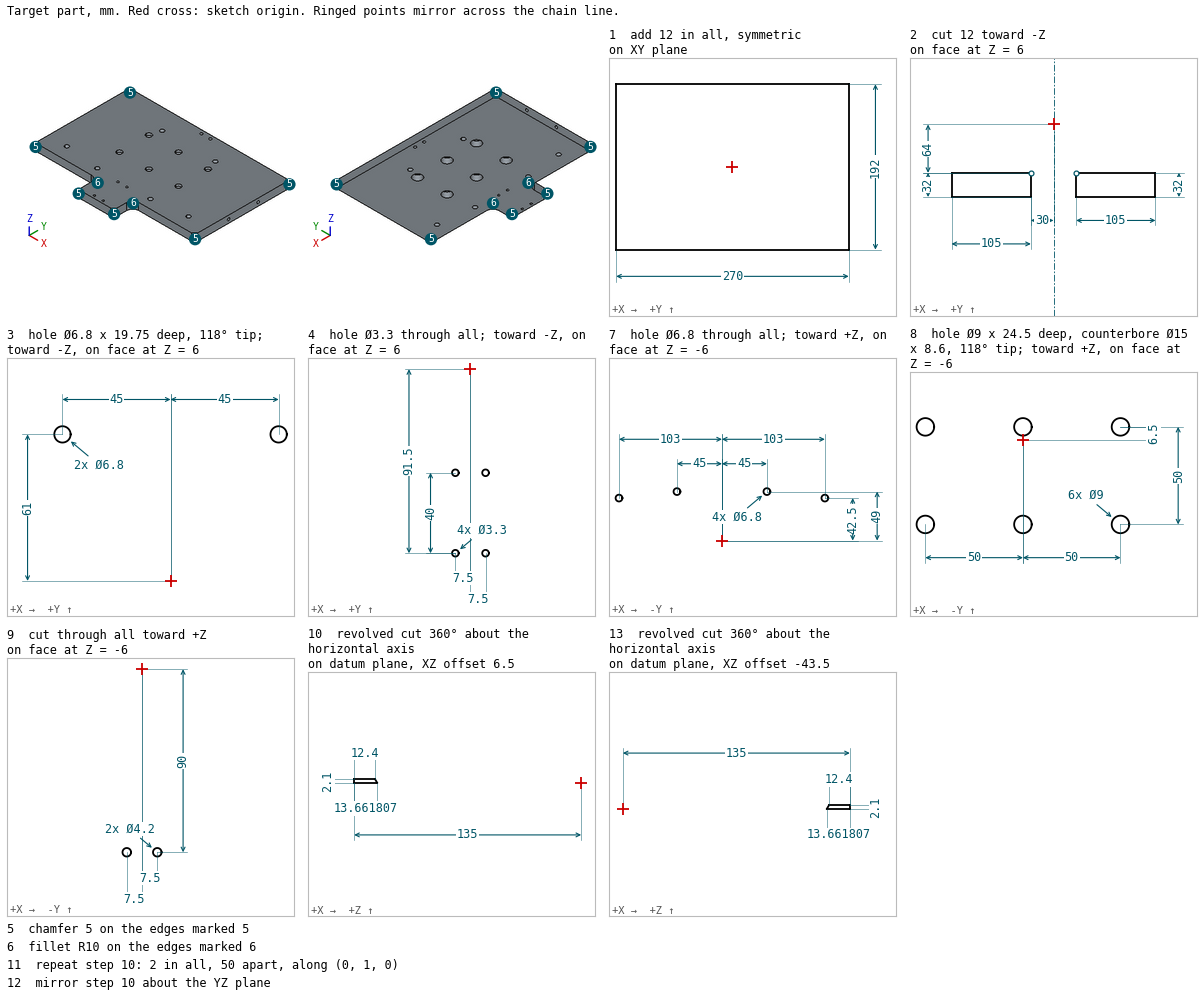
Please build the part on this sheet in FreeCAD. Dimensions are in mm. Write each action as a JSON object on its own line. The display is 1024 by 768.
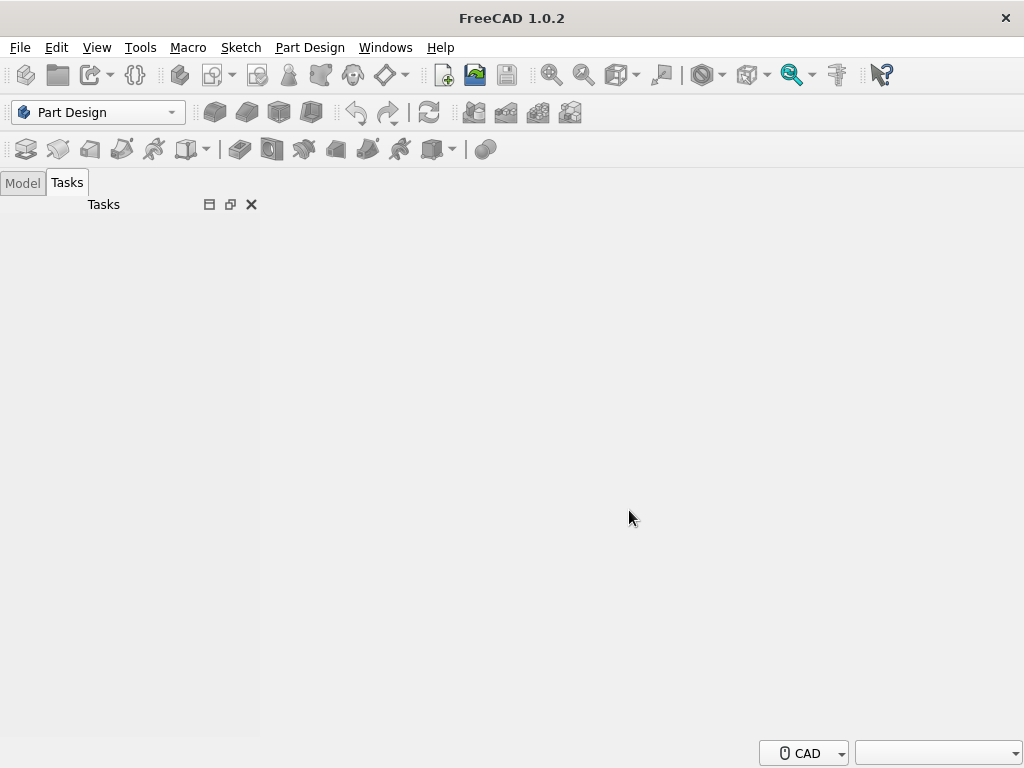
{"action": "key", "text": "ctrl+n"}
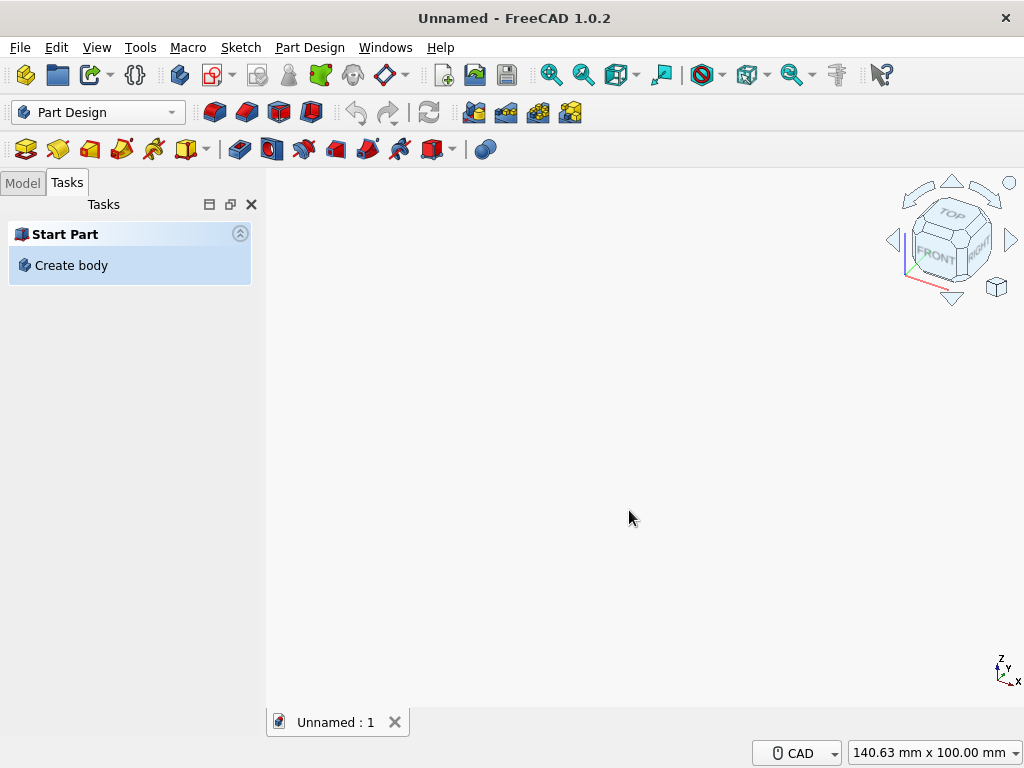
{"action": "left_click", "coordinate": [212, 76]}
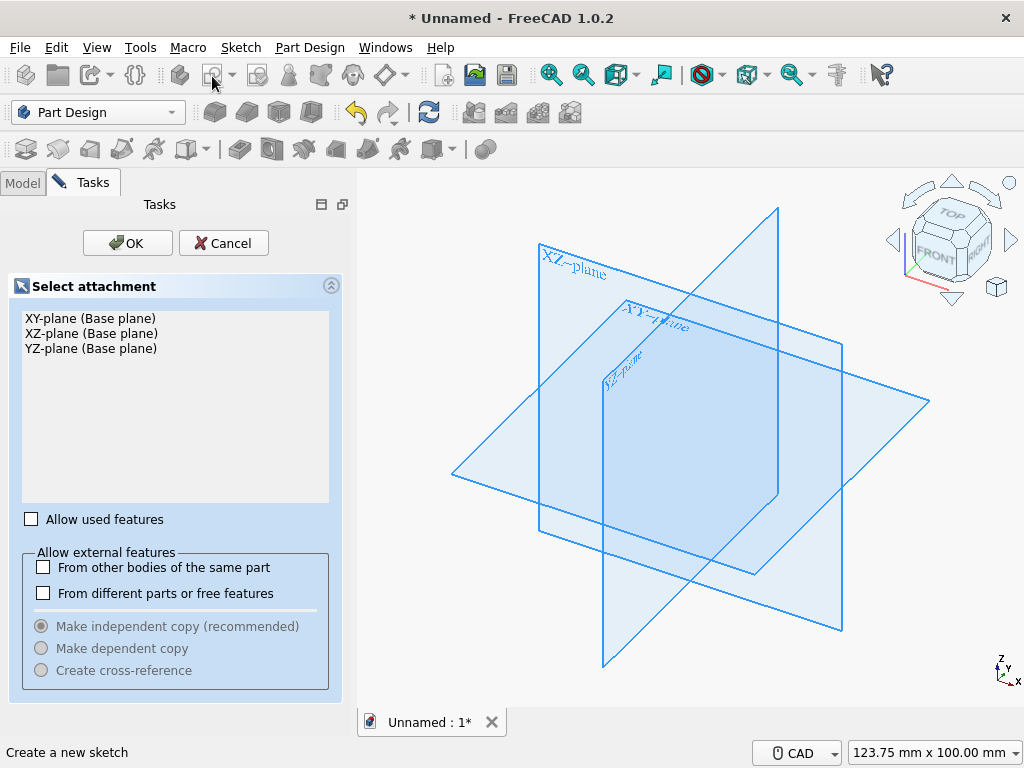
{"action": "left_click", "coordinate": [82, 318]}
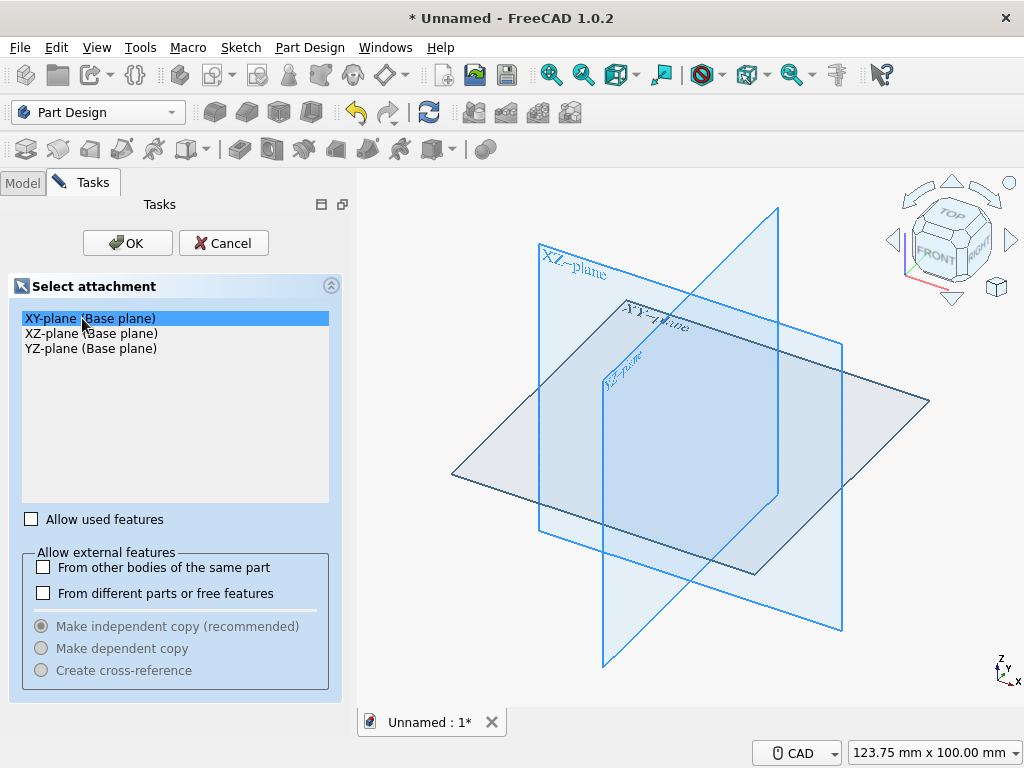
{"action": "left_click", "coordinate": [128, 243]}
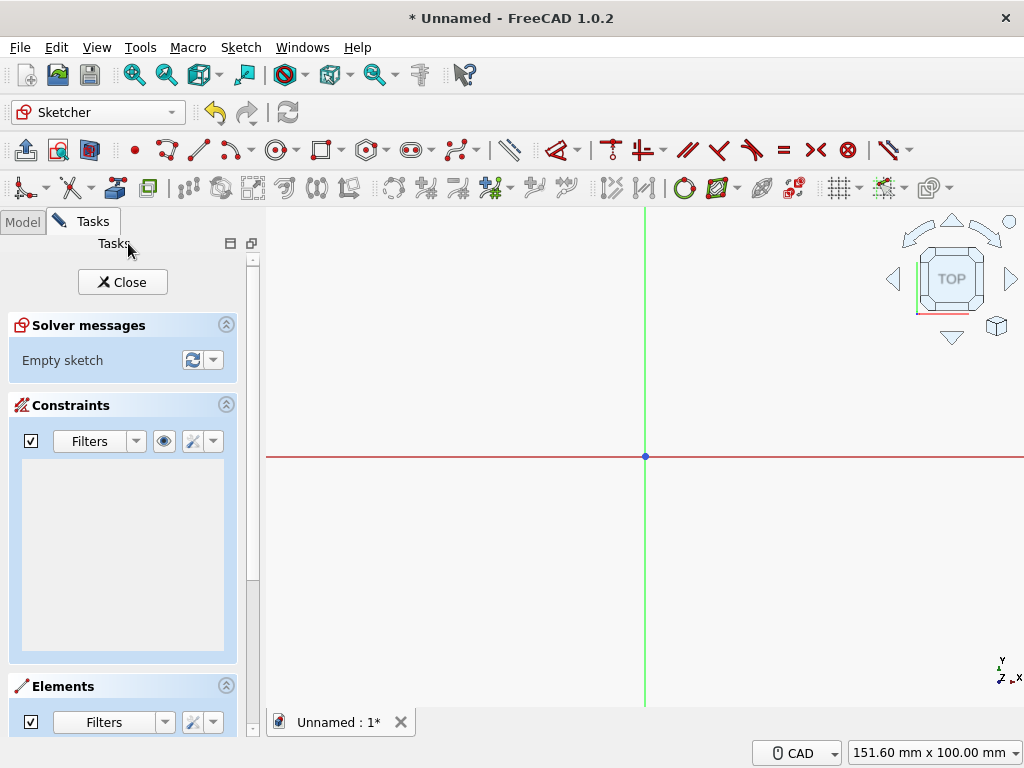
{"action": "scroll", "coordinate": [547, 457], "scroll_direction": "down", "scroll_amount": 6}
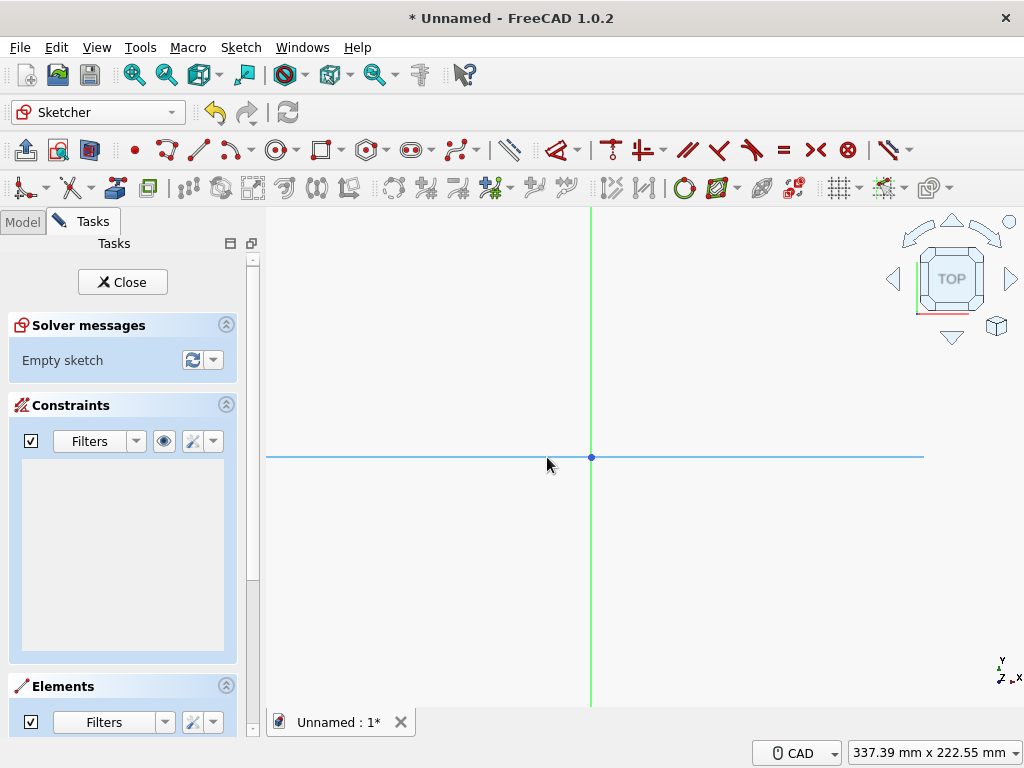
{"action": "key", "text": "g v"}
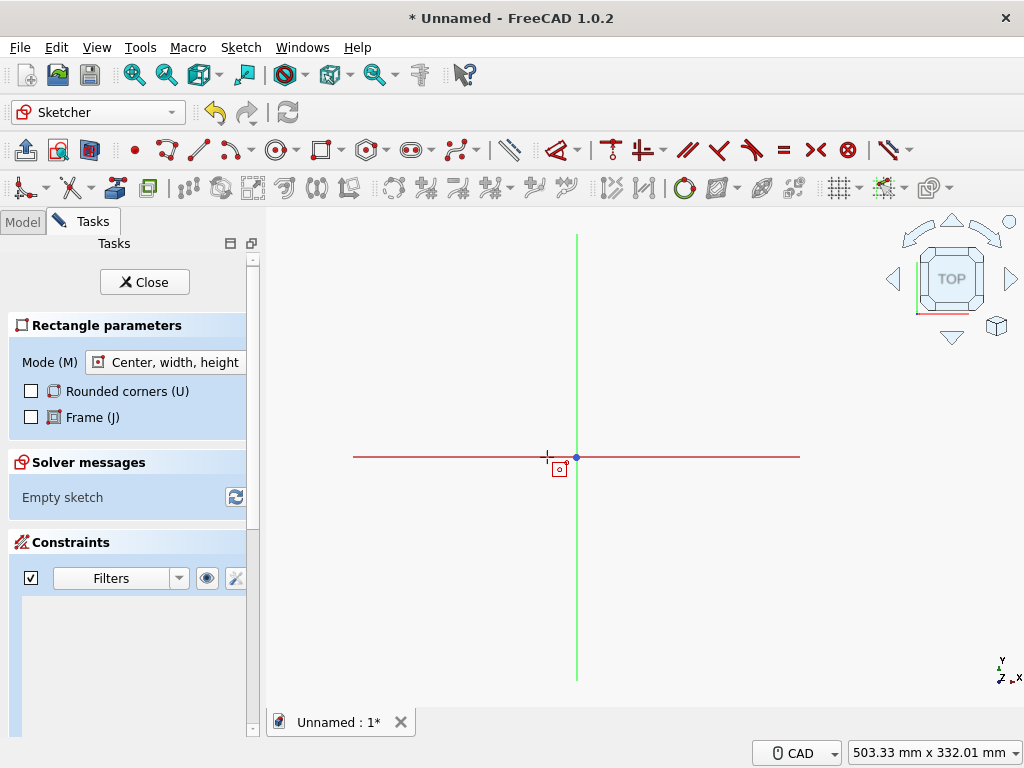
{"action": "left_click", "coordinate": [577, 457]}
{"action": "mouse_move", "coordinate": [780, 313]}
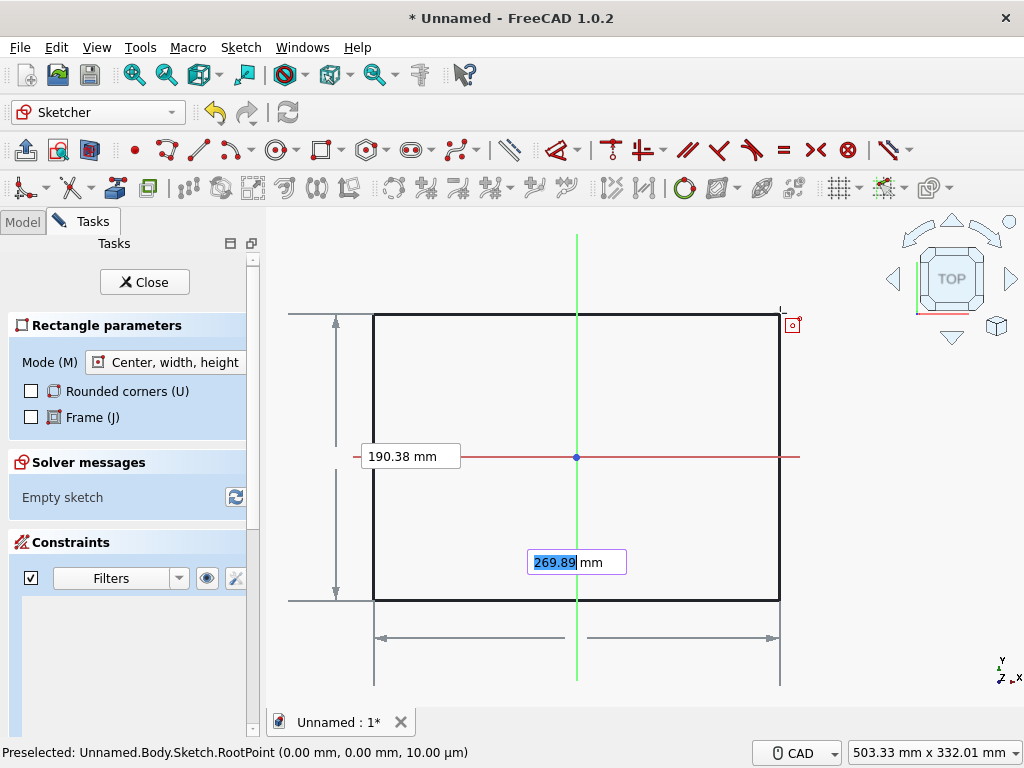
{"action": "type", "text": "270"}
{"action": "key", "text": "Tab"}
{"action": "type", "text": "192"}
{"action": "key", "text": "Return"}
{"action": "key", "text": "Escape"}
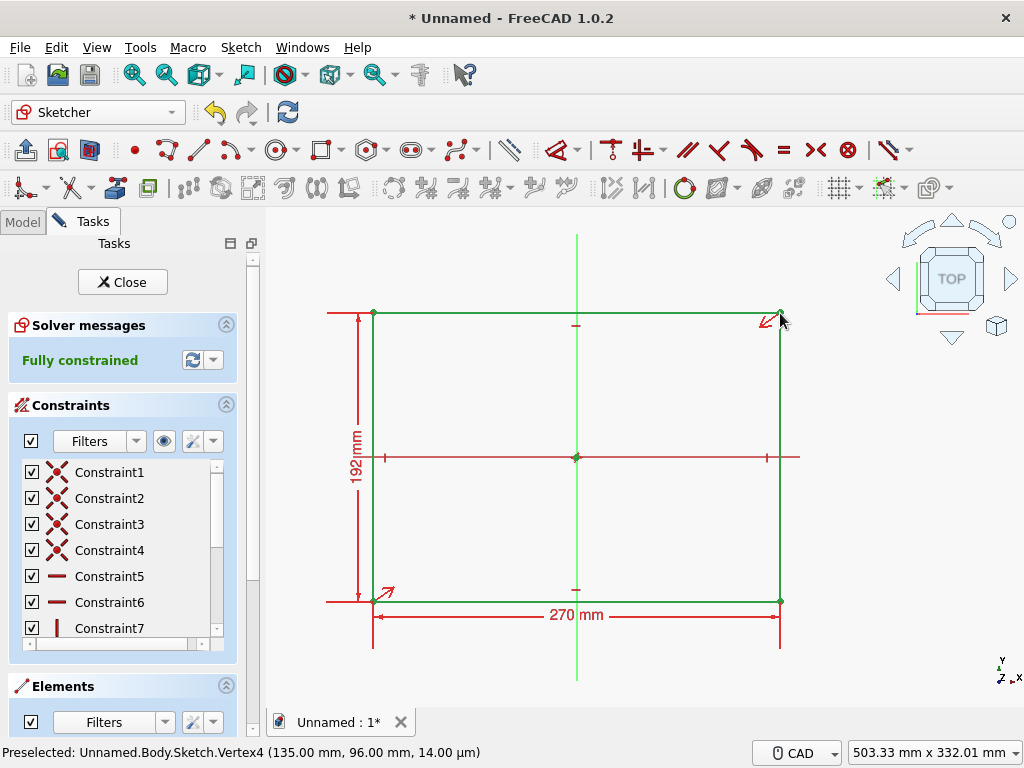
{"action": "left_click", "coordinate": [123, 282]}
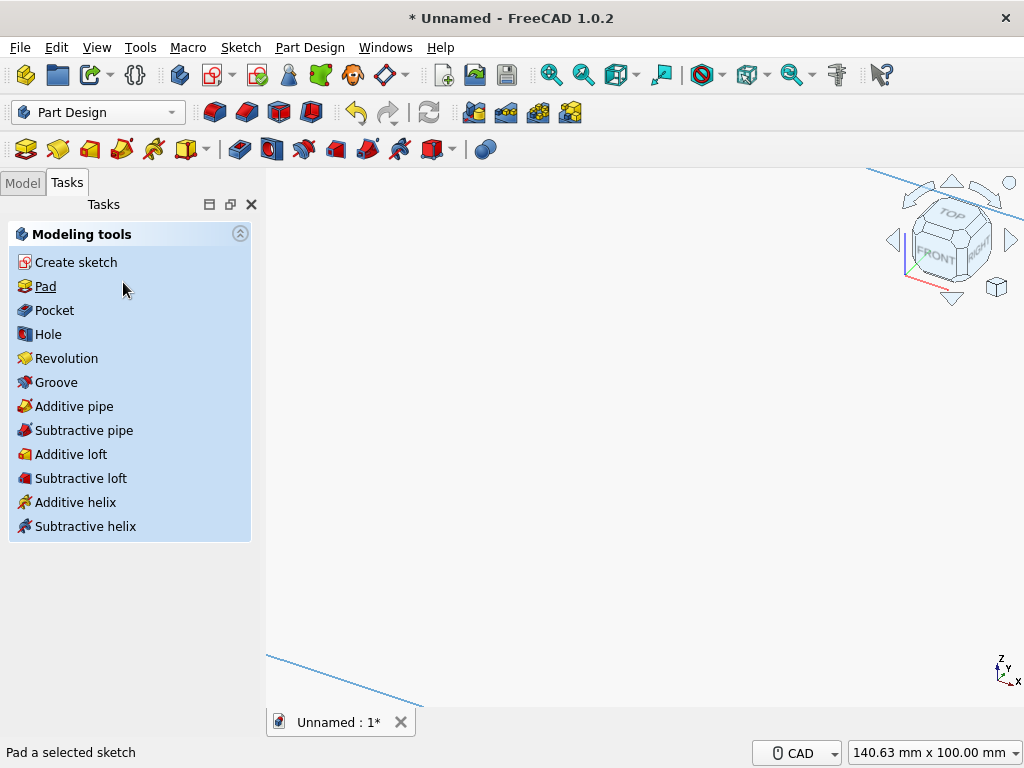
{"action": "left_click", "coordinate": [26, 150]}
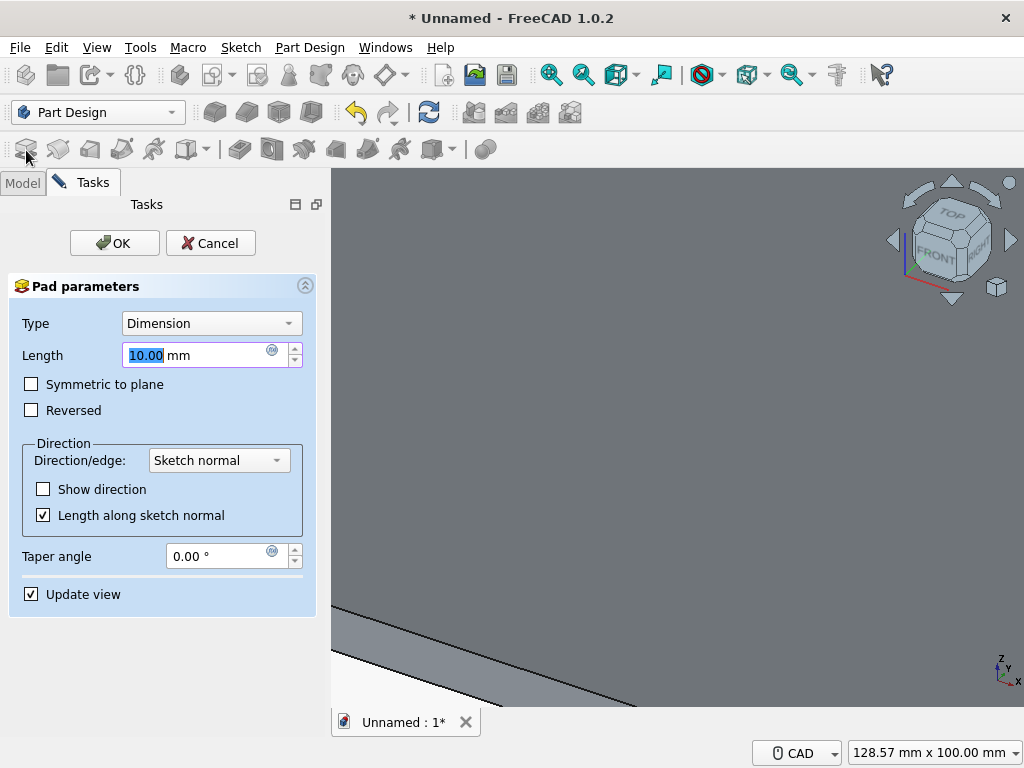
{"action": "type", "text": "12"}
{"action": "key", "text": "Tab"}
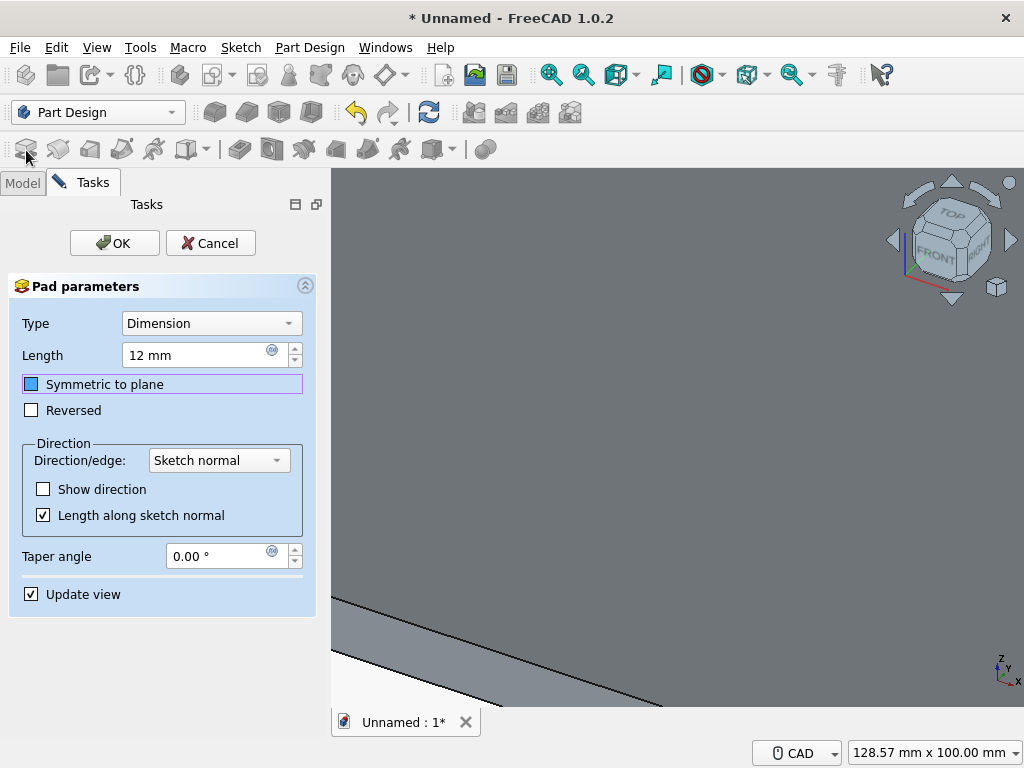
{"action": "left_click", "coordinate": [30, 384]}